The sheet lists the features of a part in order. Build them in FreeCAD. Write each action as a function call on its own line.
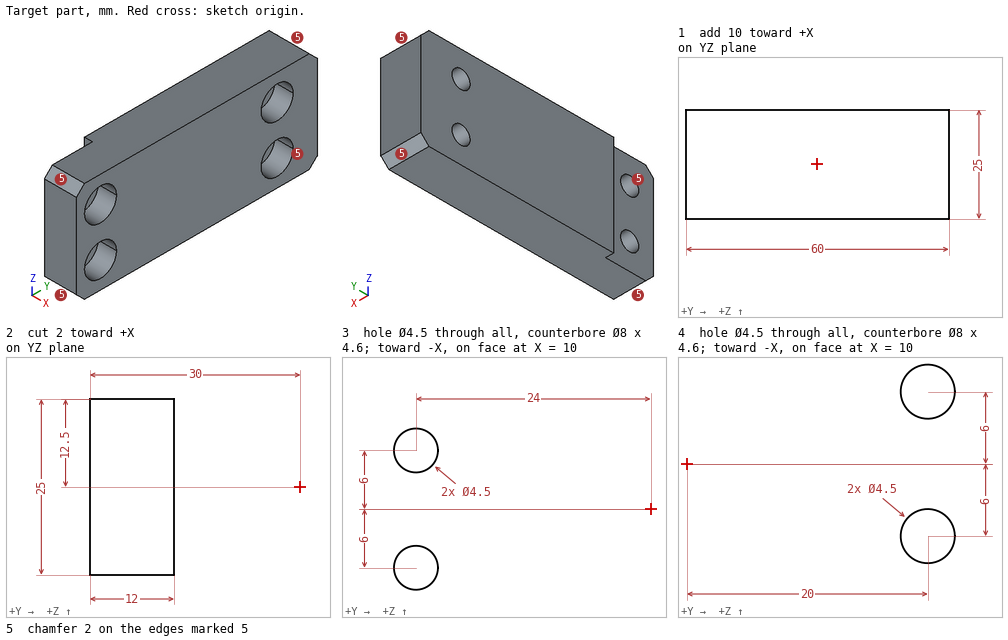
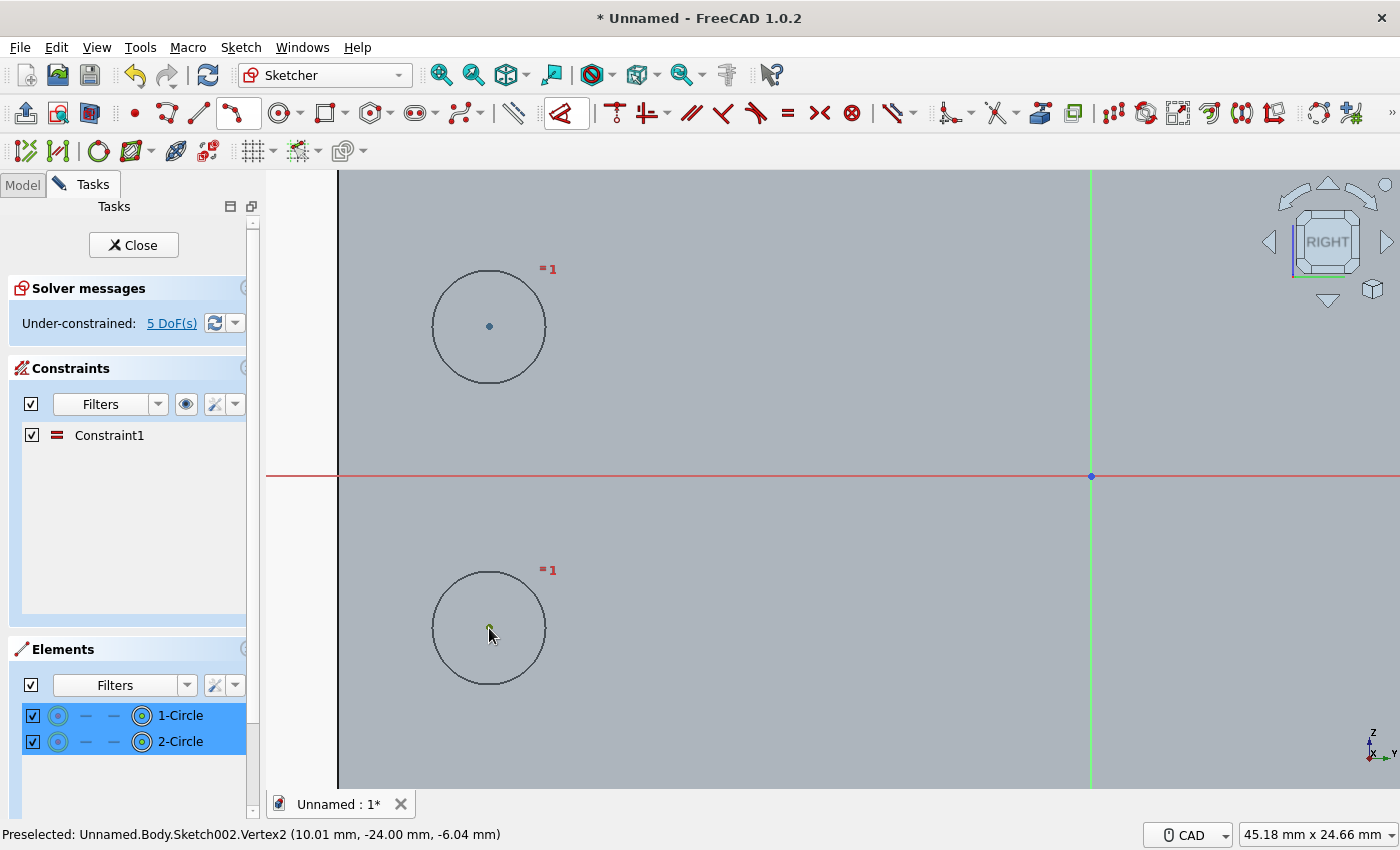
key(v)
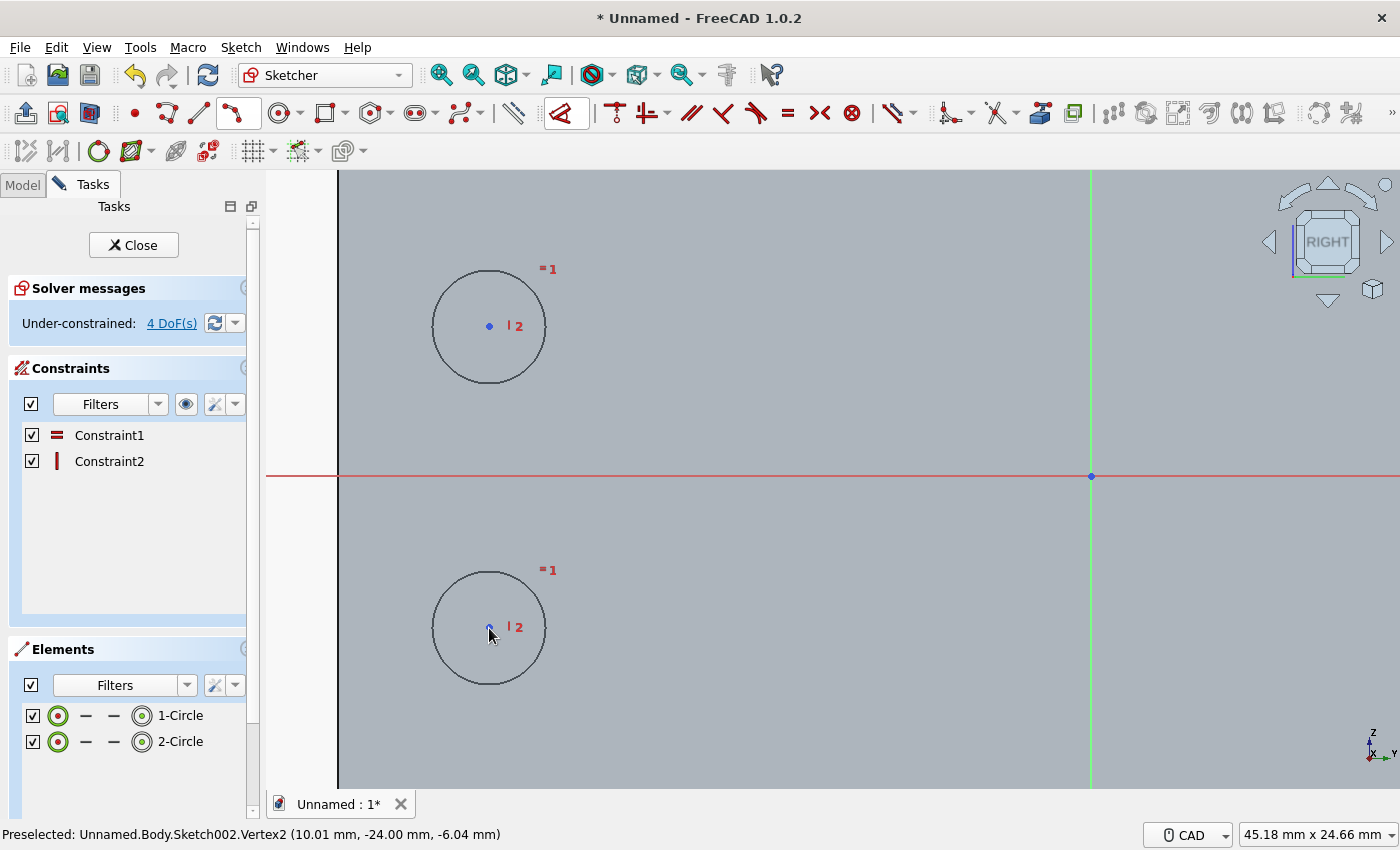
click(529, 287)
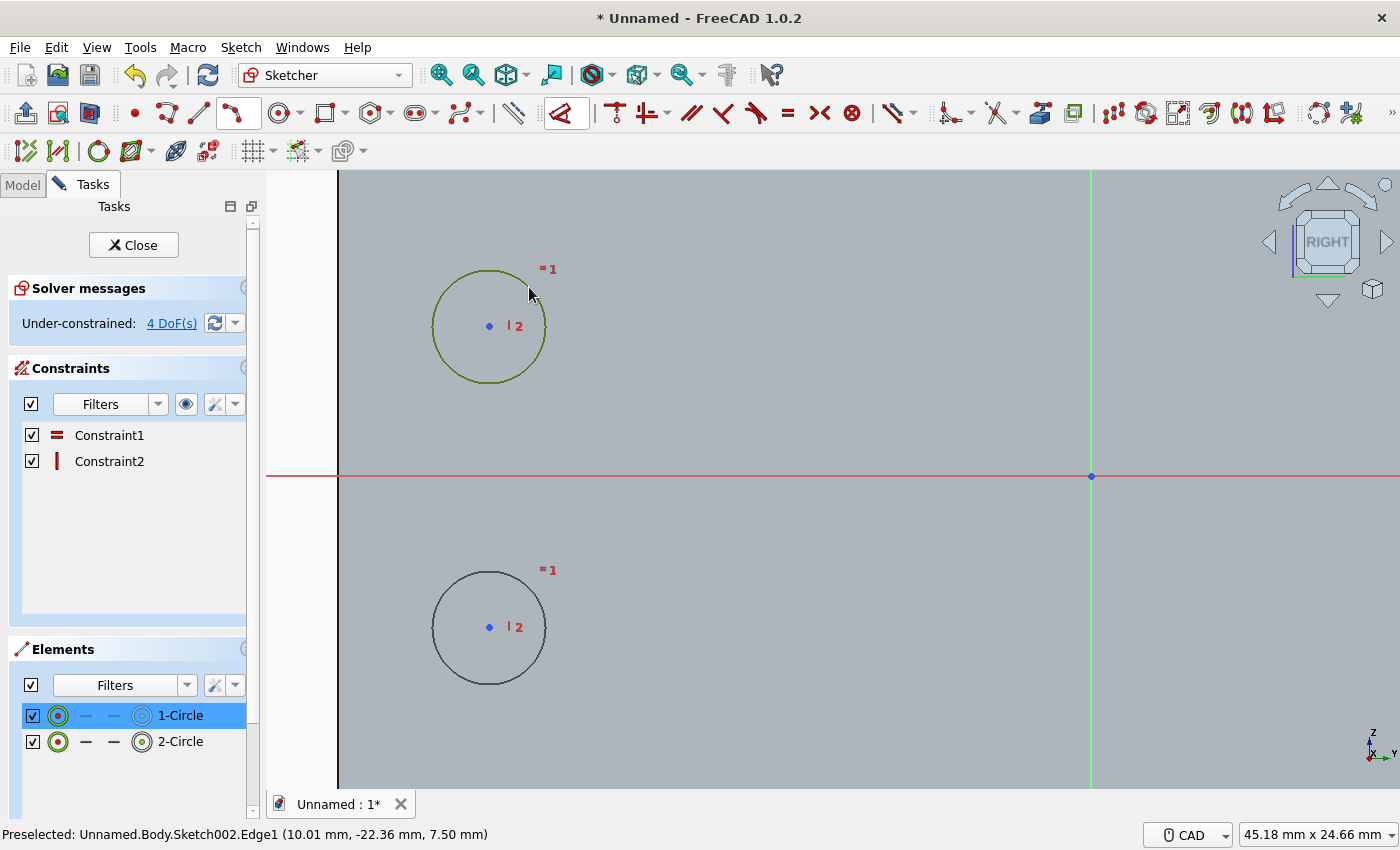
click(584, 114)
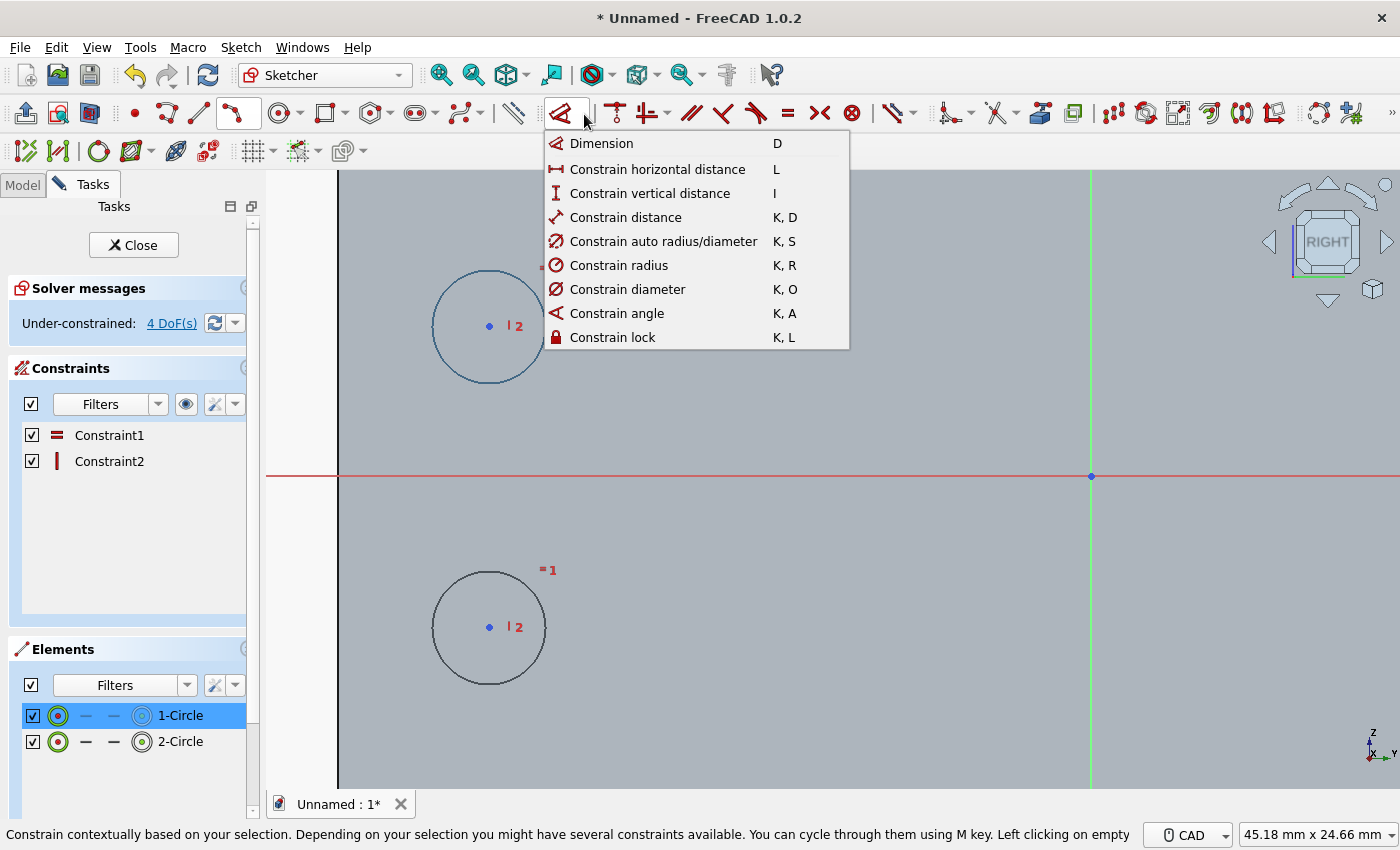
click(697, 289)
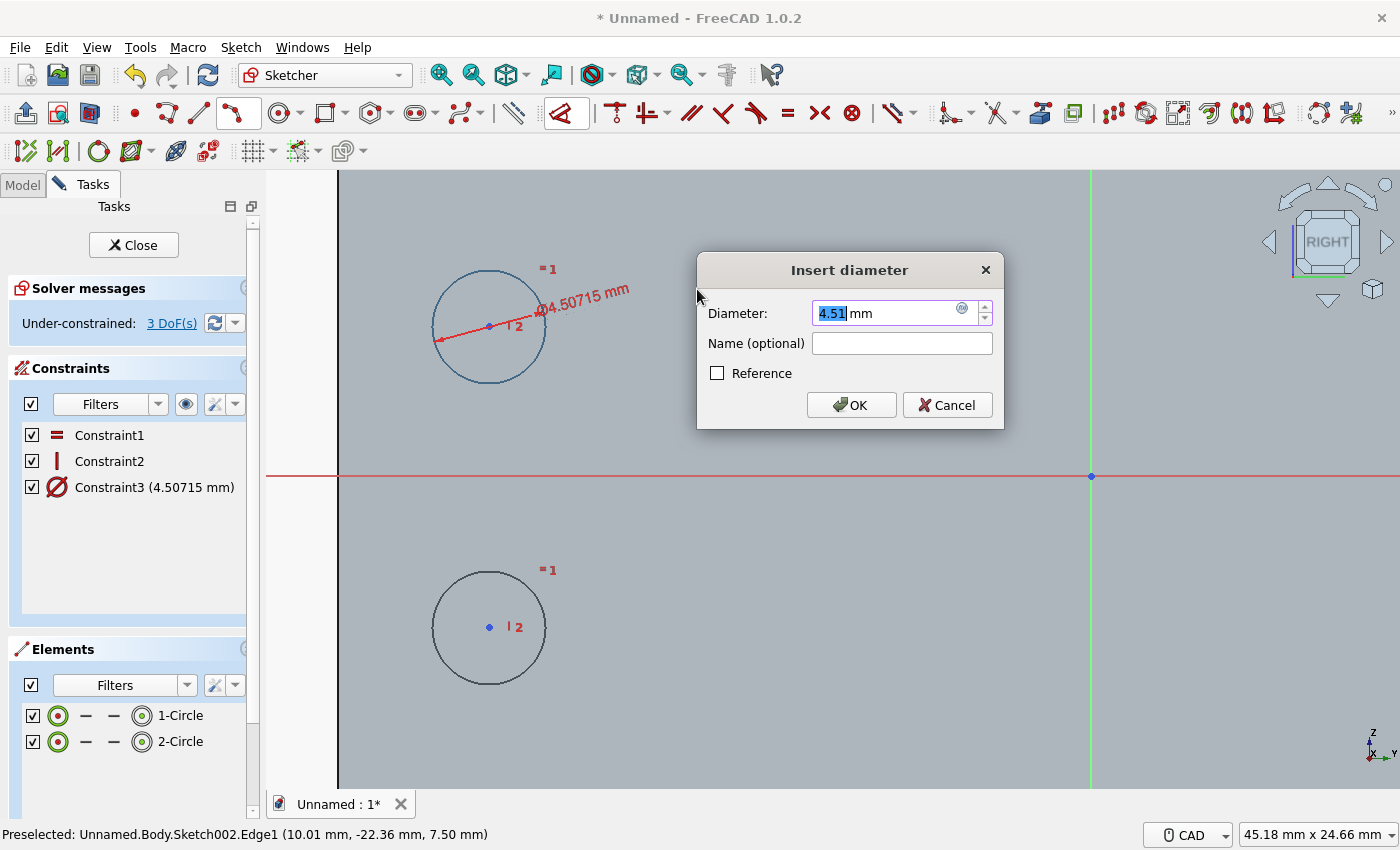
text(4.5)
key(Return)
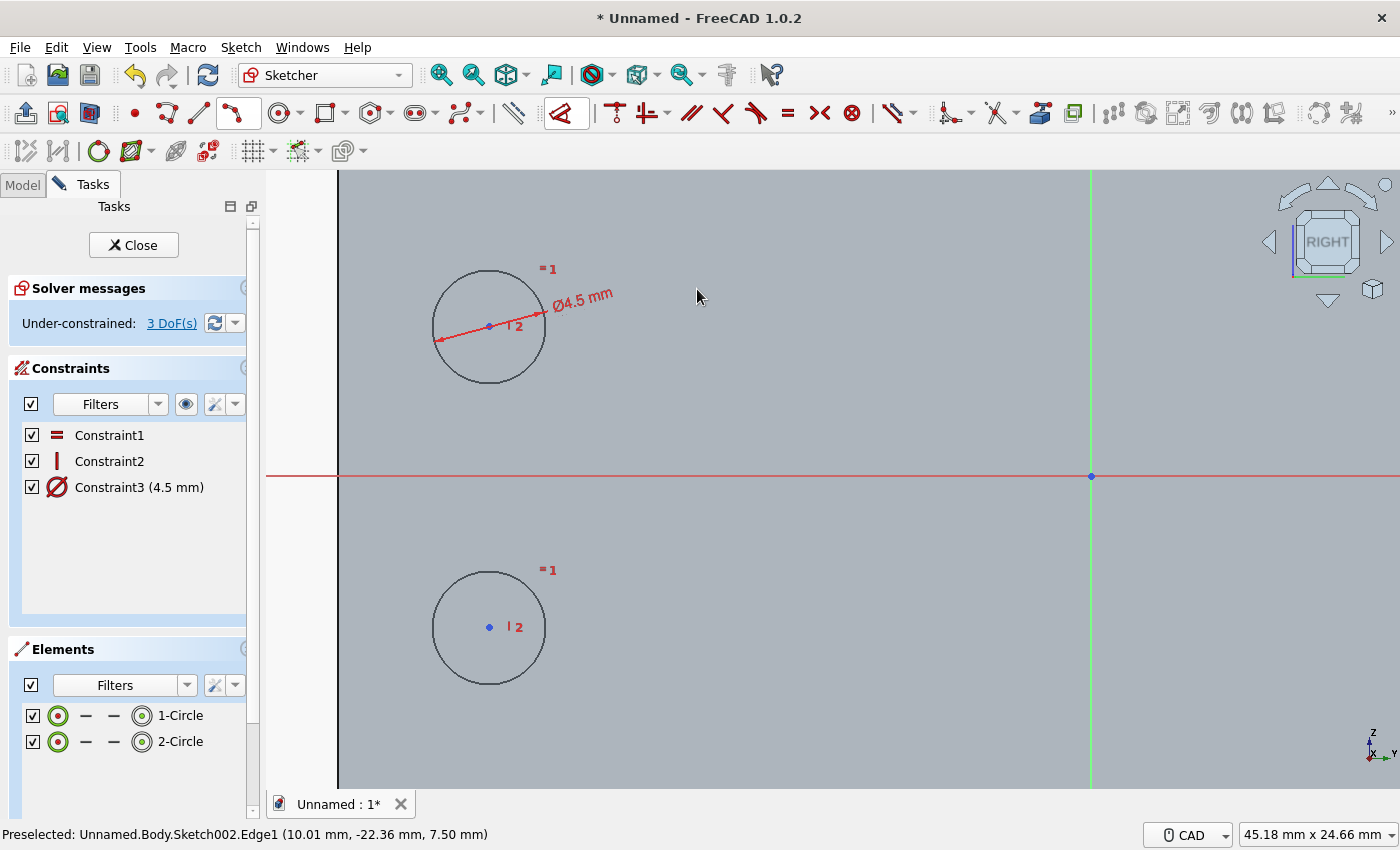
click(489, 327)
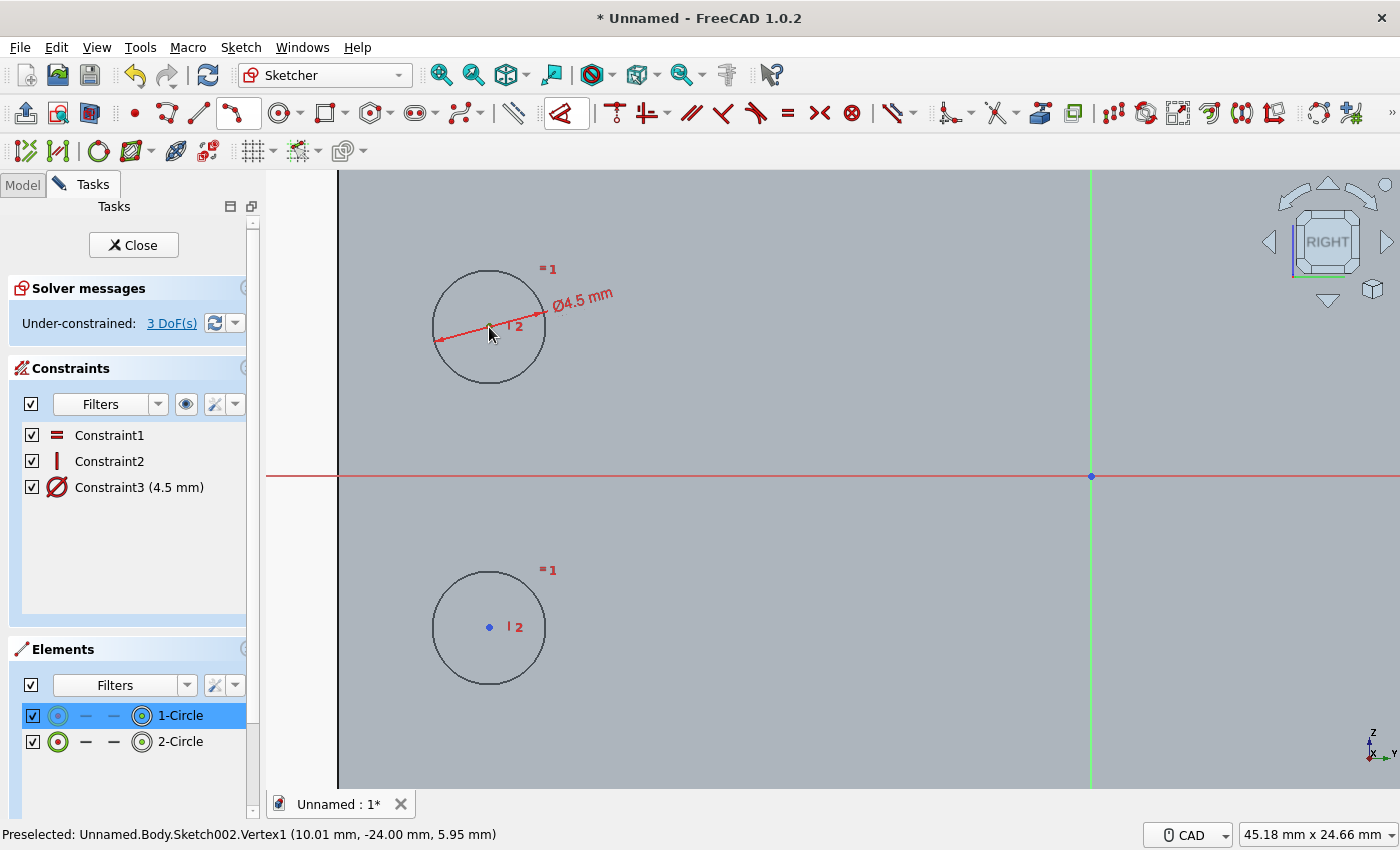
key(i)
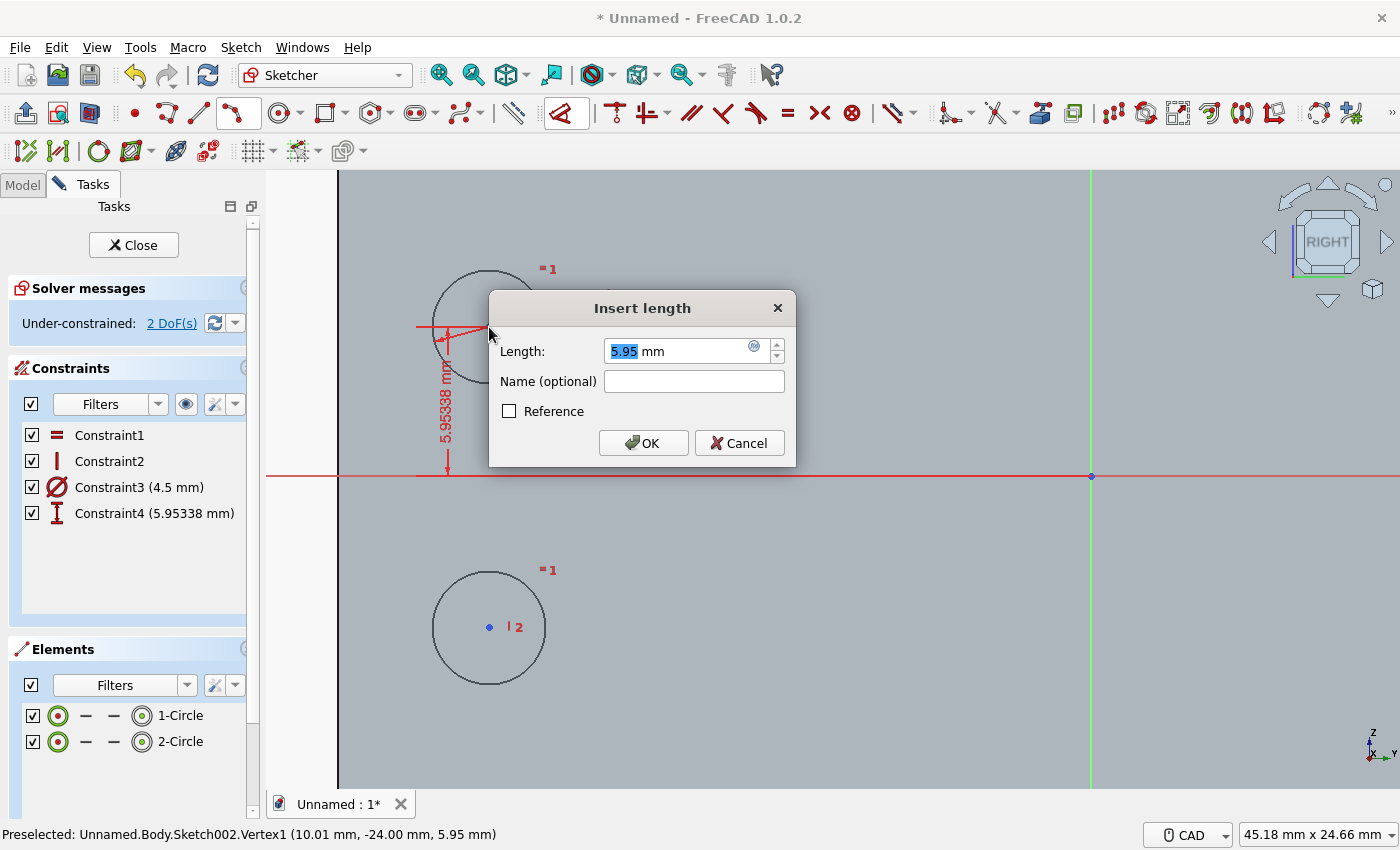
text(6)
key(Return)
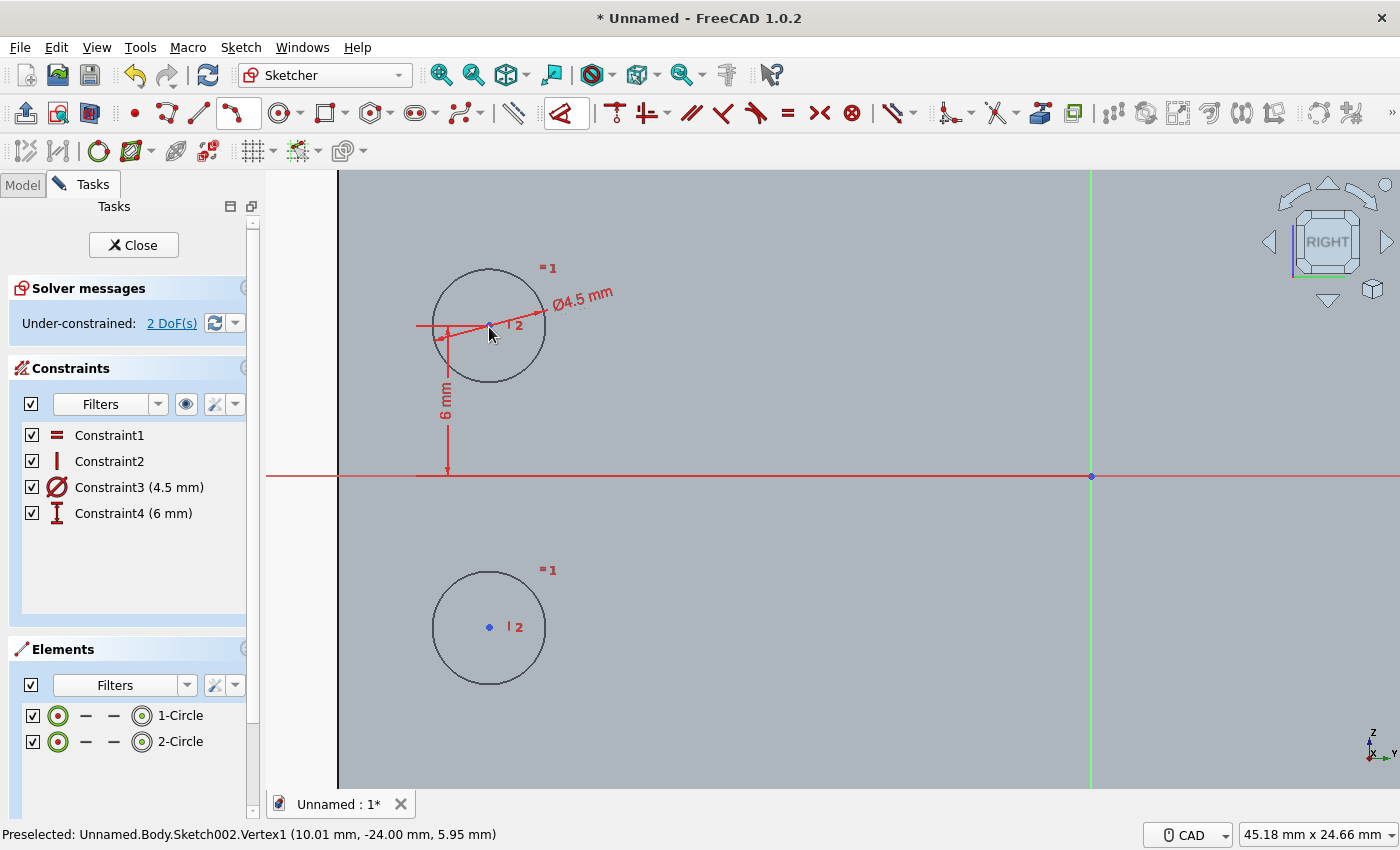
click(489, 628)